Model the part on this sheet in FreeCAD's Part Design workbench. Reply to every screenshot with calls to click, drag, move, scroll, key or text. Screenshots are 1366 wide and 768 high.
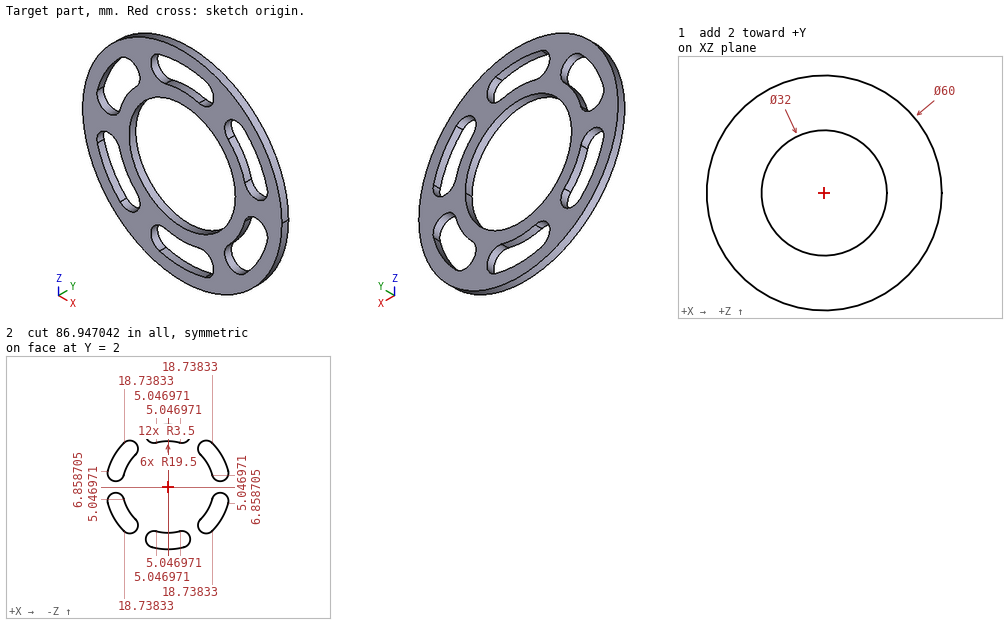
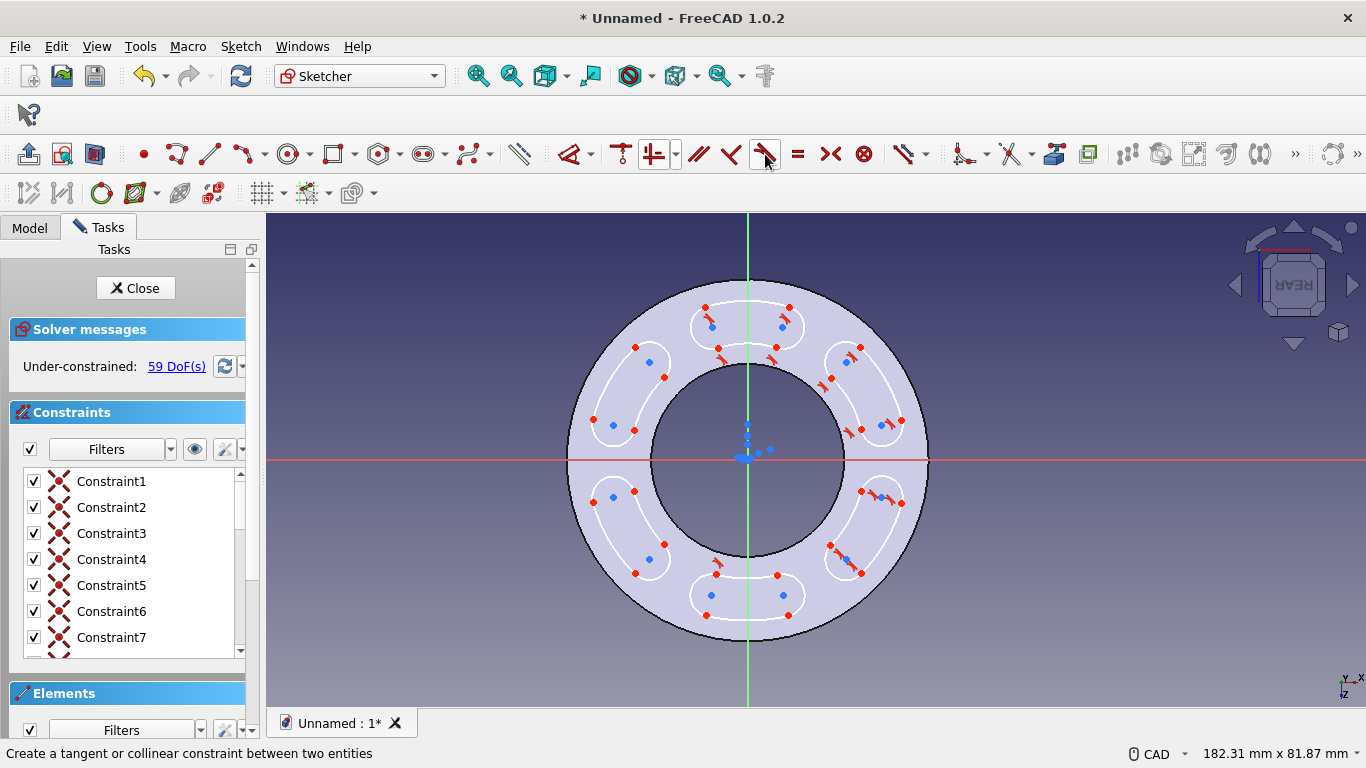
click(735, 578)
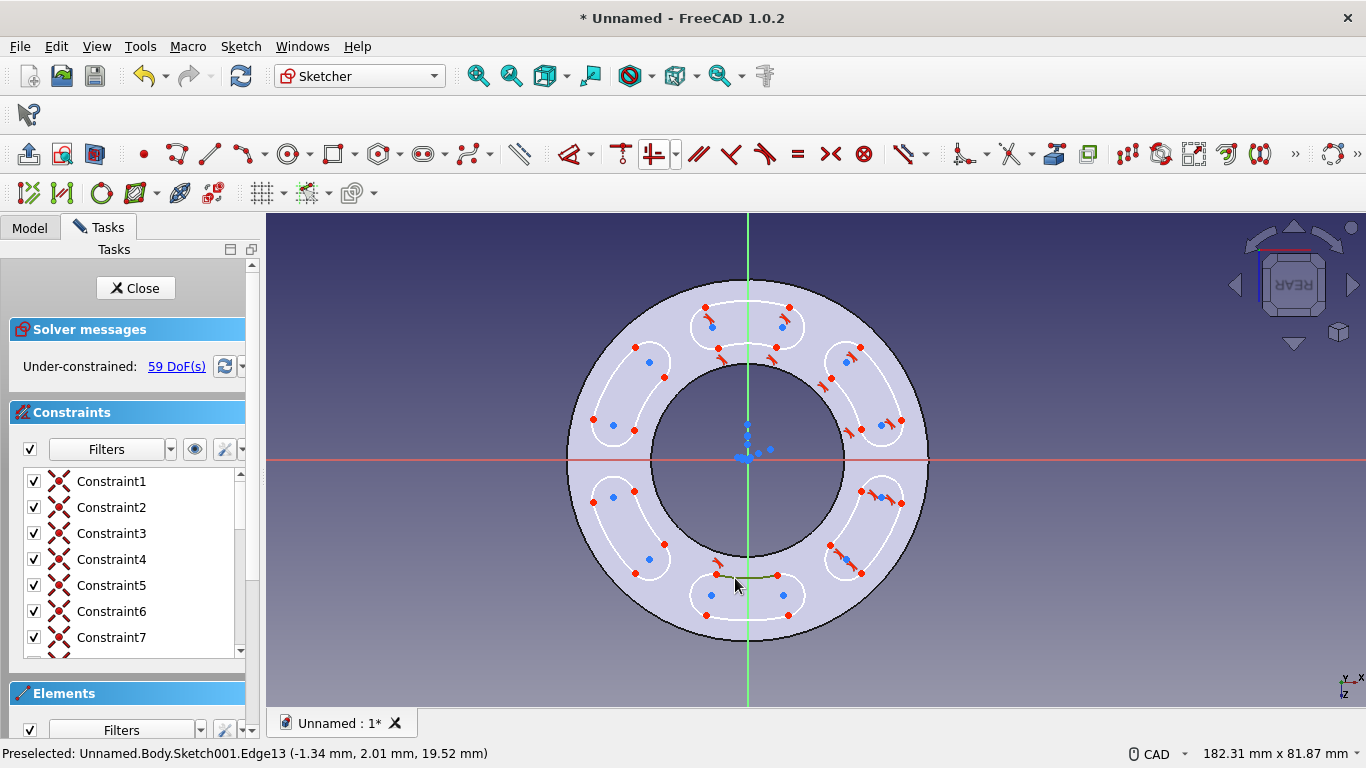
click(803, 603)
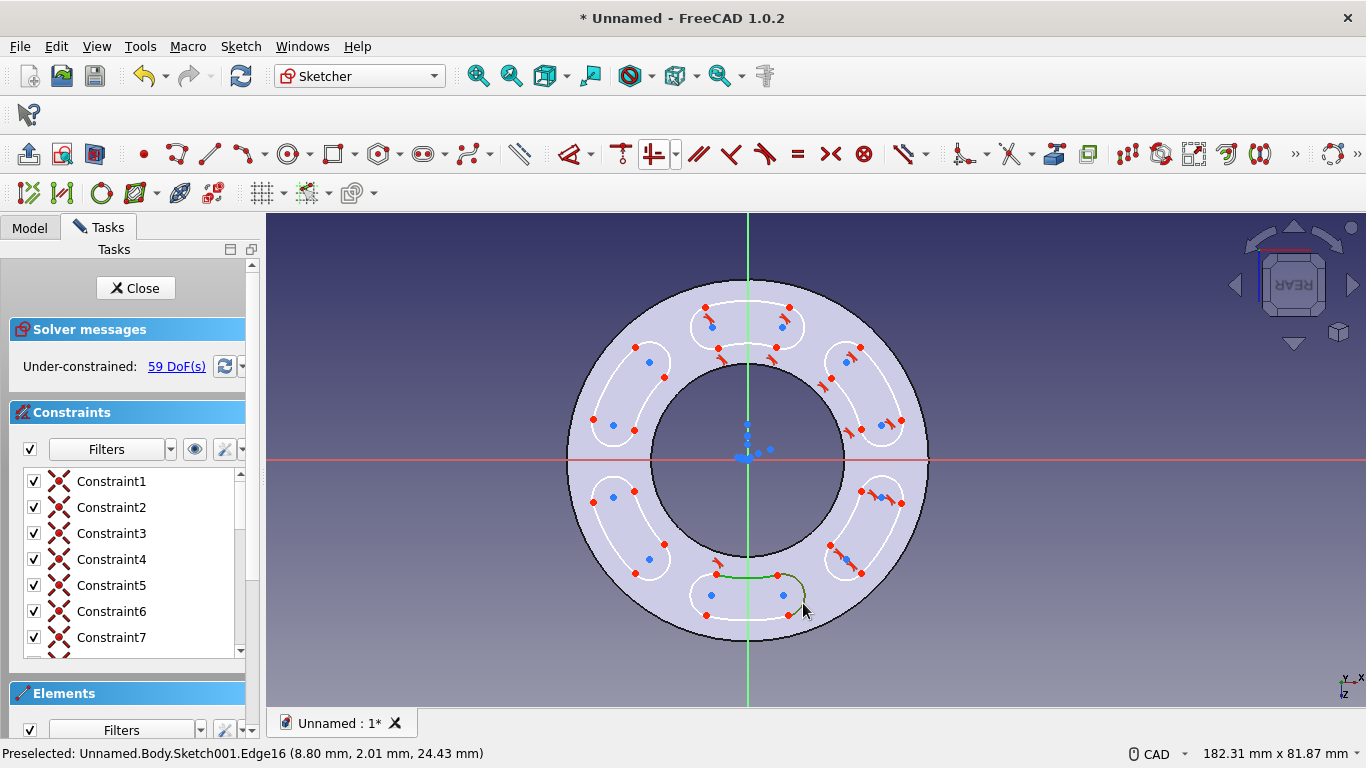
click(765, 154)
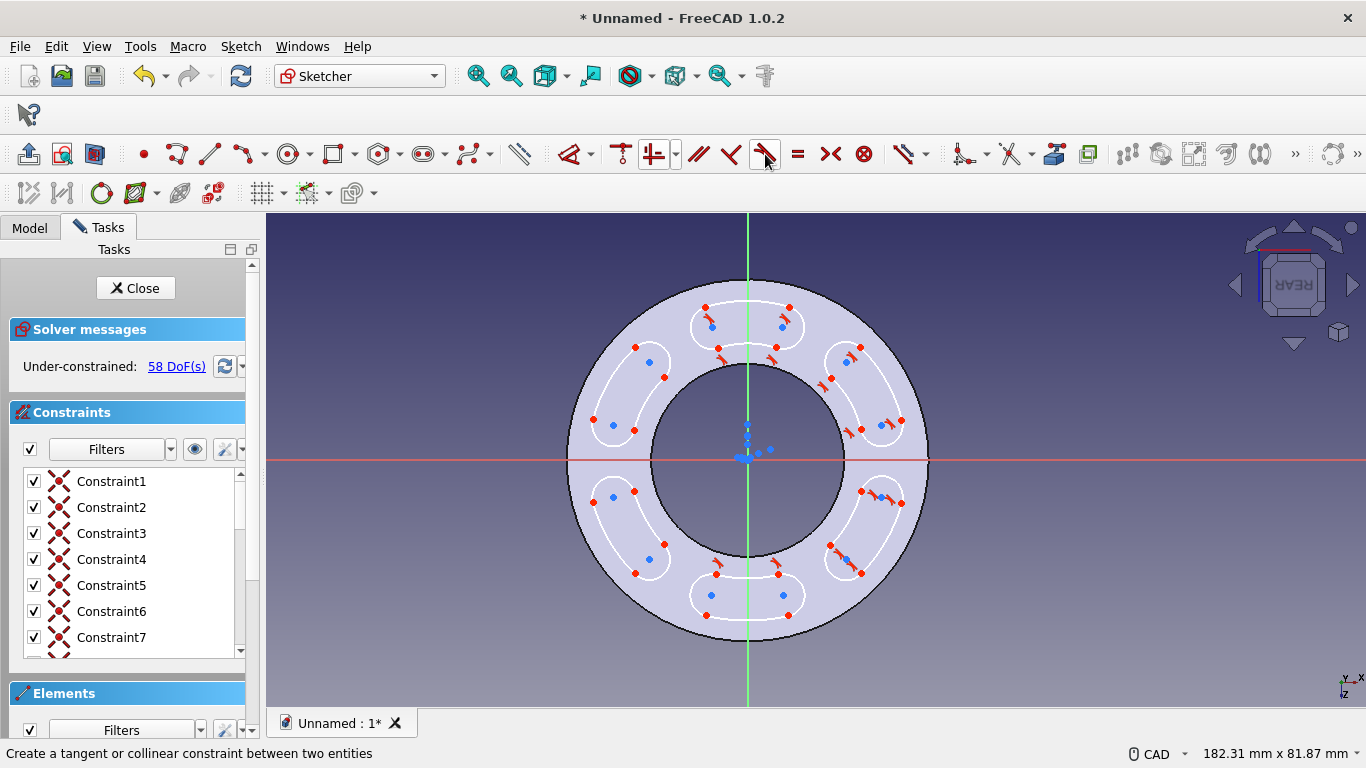
click(698, 579)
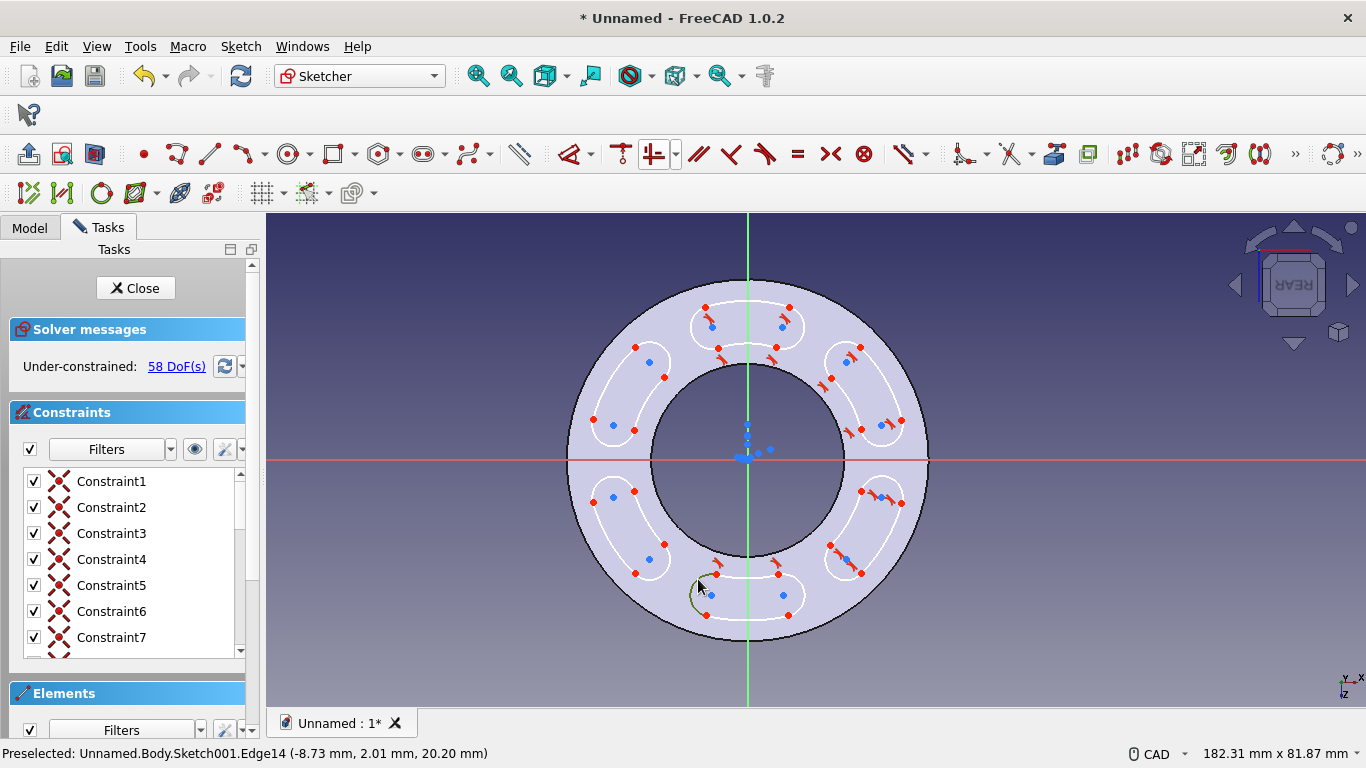
click(731, 620)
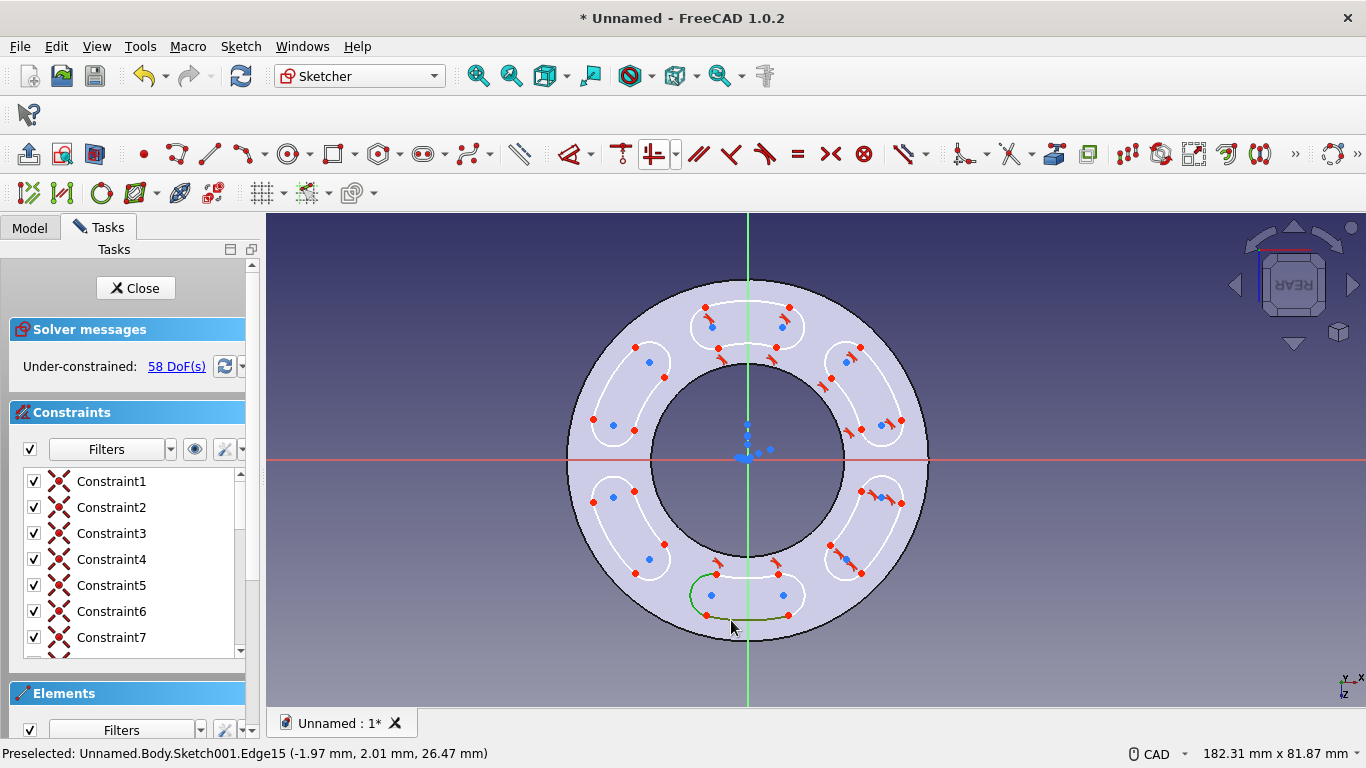
click(765, 154)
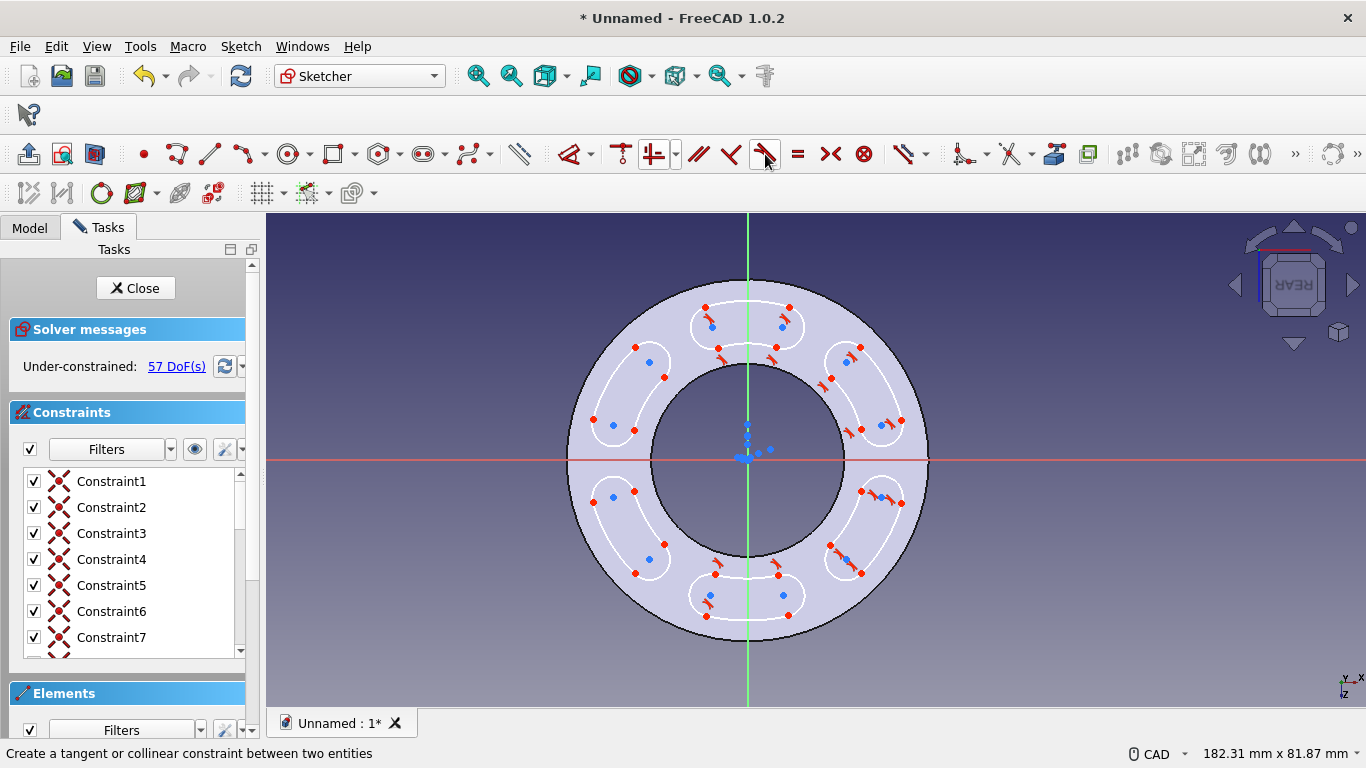
click(731, 620)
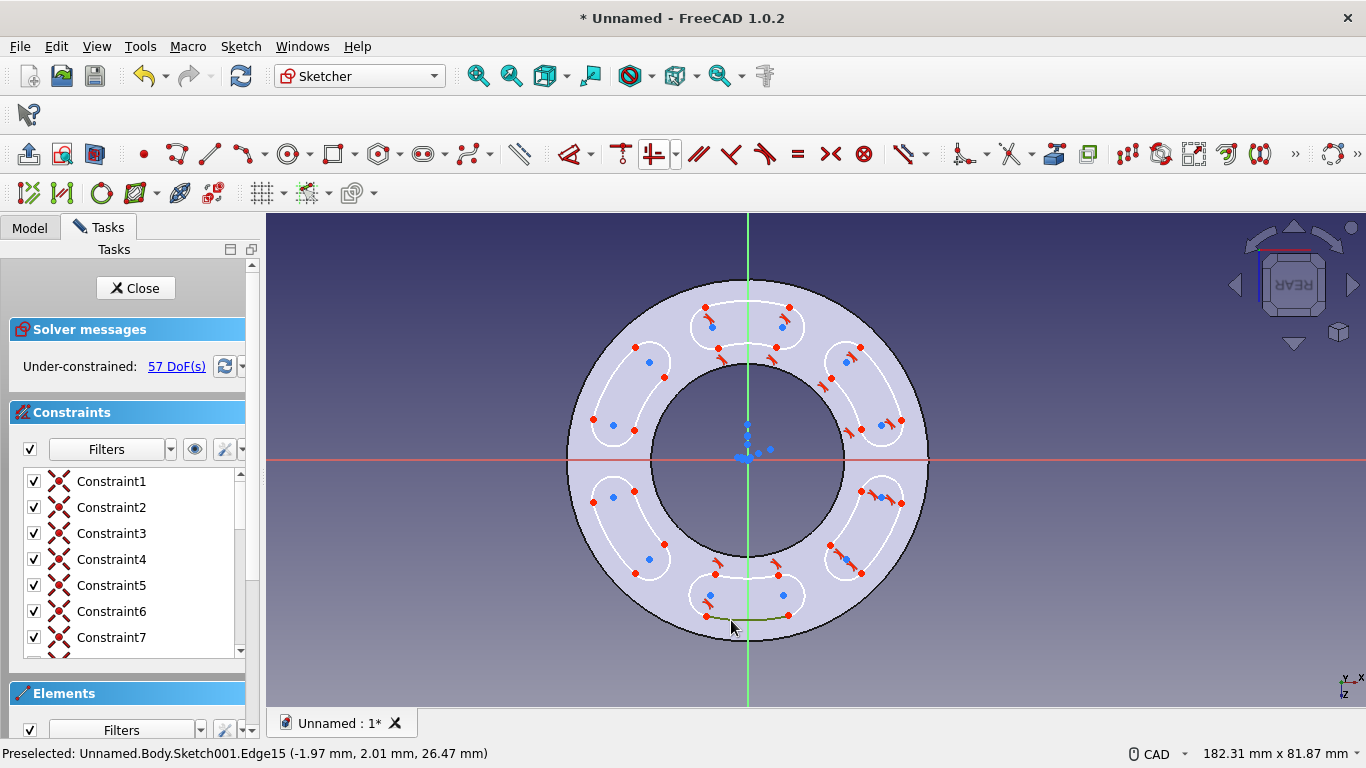
click(803, 603)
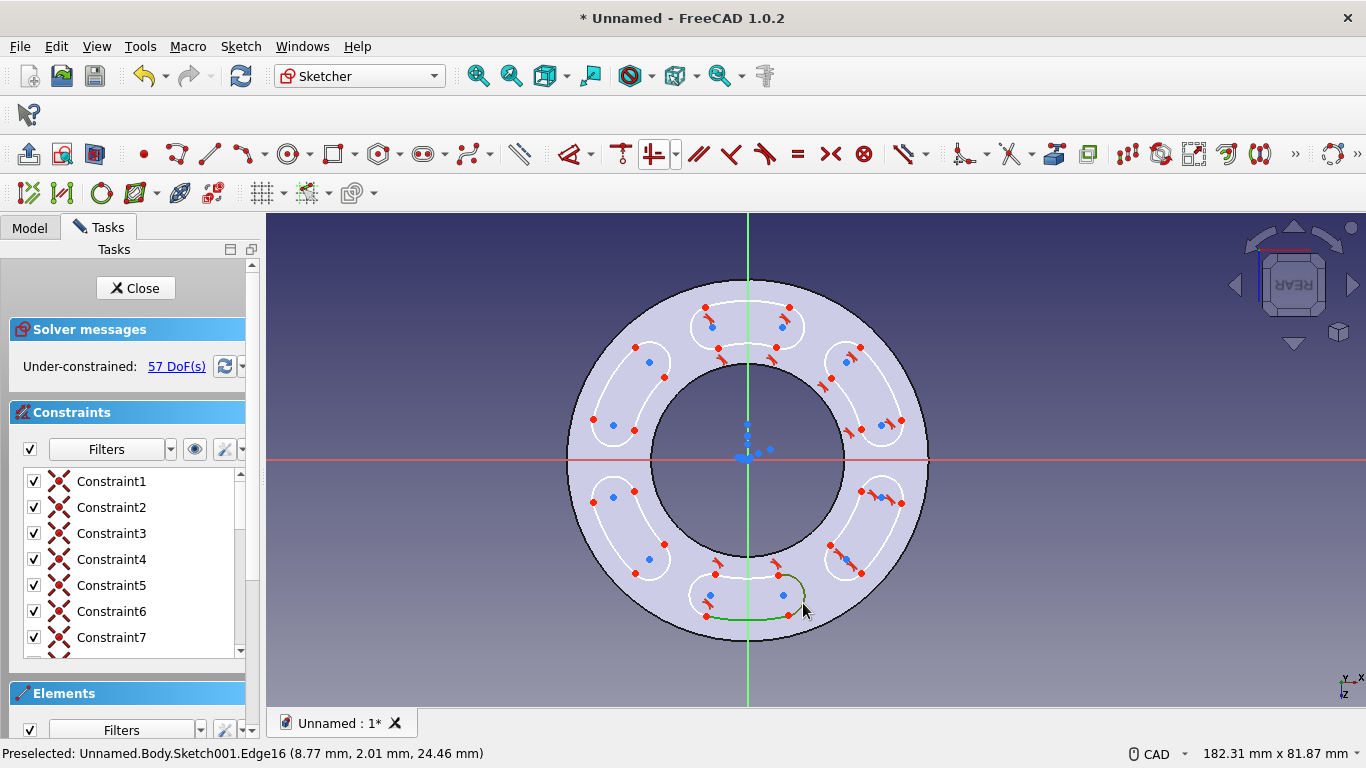
click(765, 154)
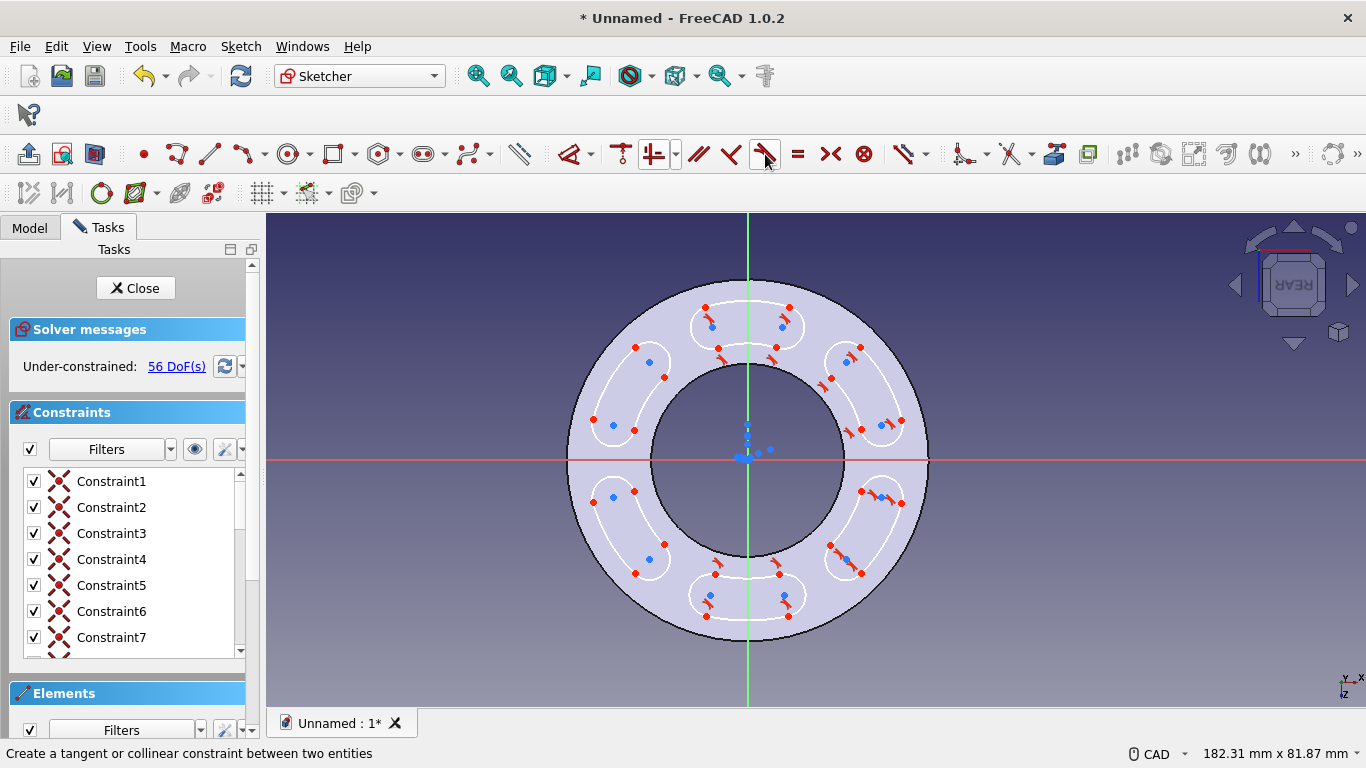
click(641, 509)